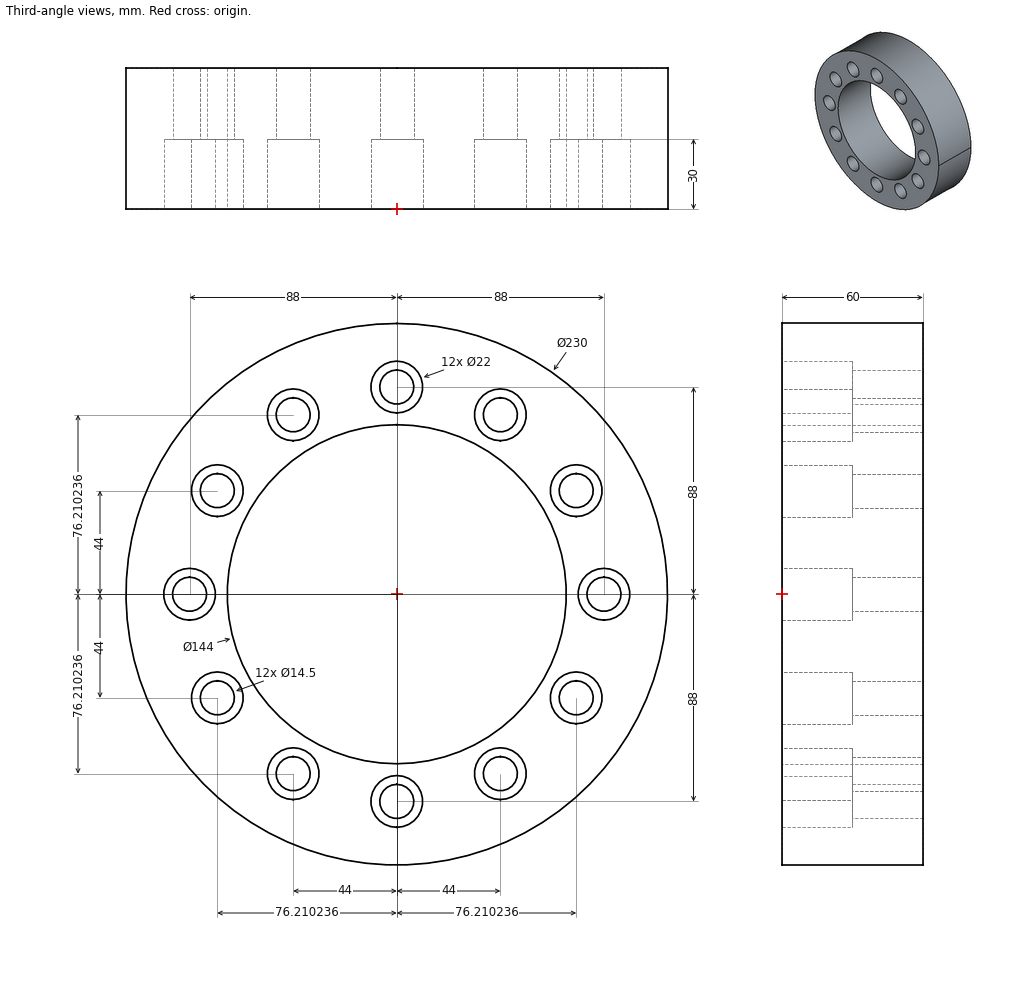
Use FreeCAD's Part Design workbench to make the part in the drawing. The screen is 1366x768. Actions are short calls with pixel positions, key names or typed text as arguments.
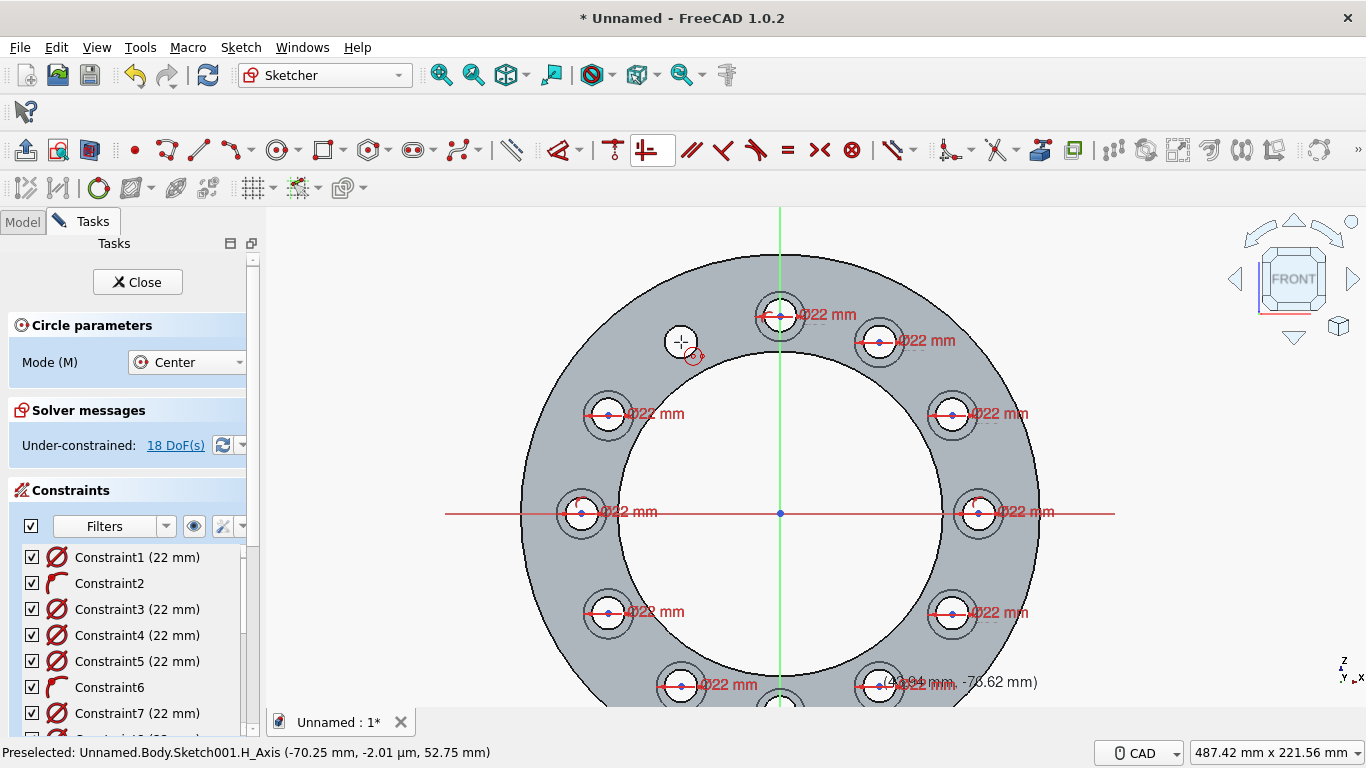
click(681, 342)
move(699, 324)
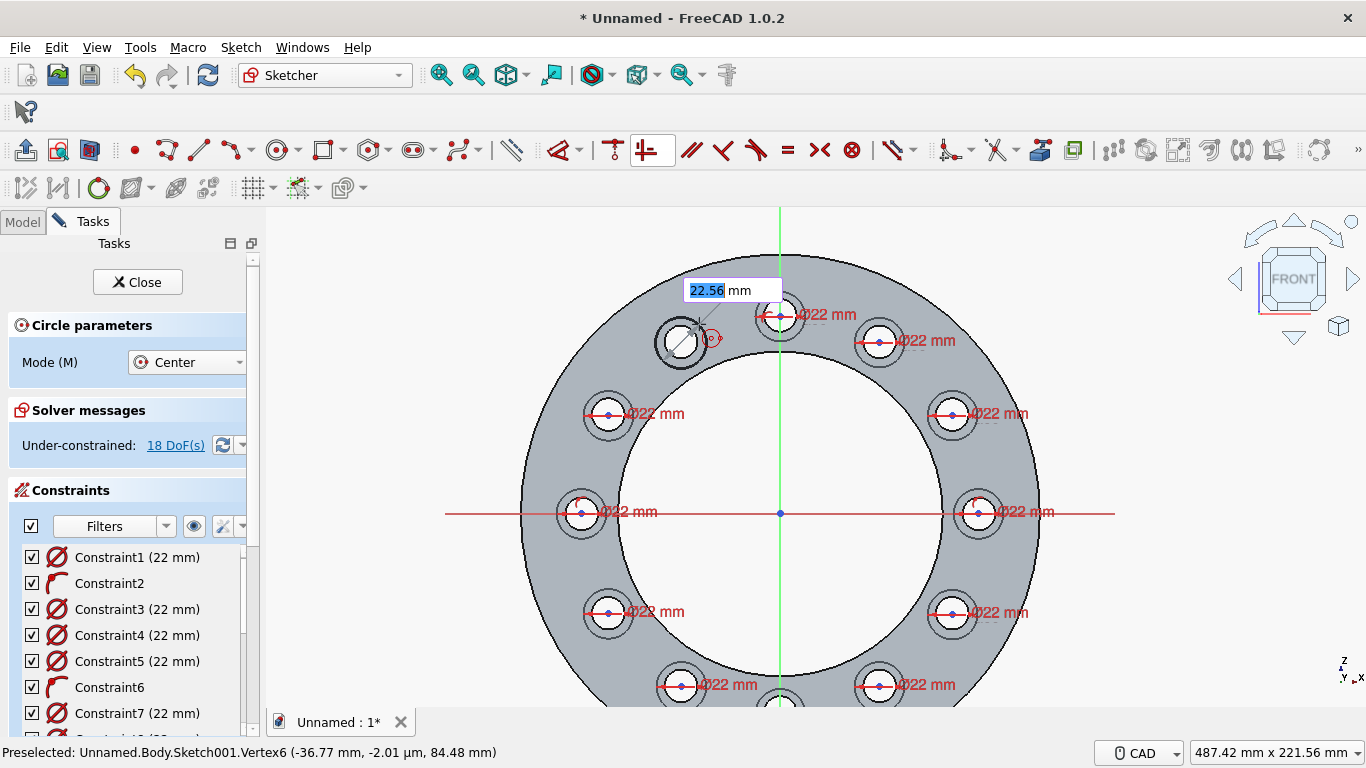
text(22)
key(Return)
key(Escape)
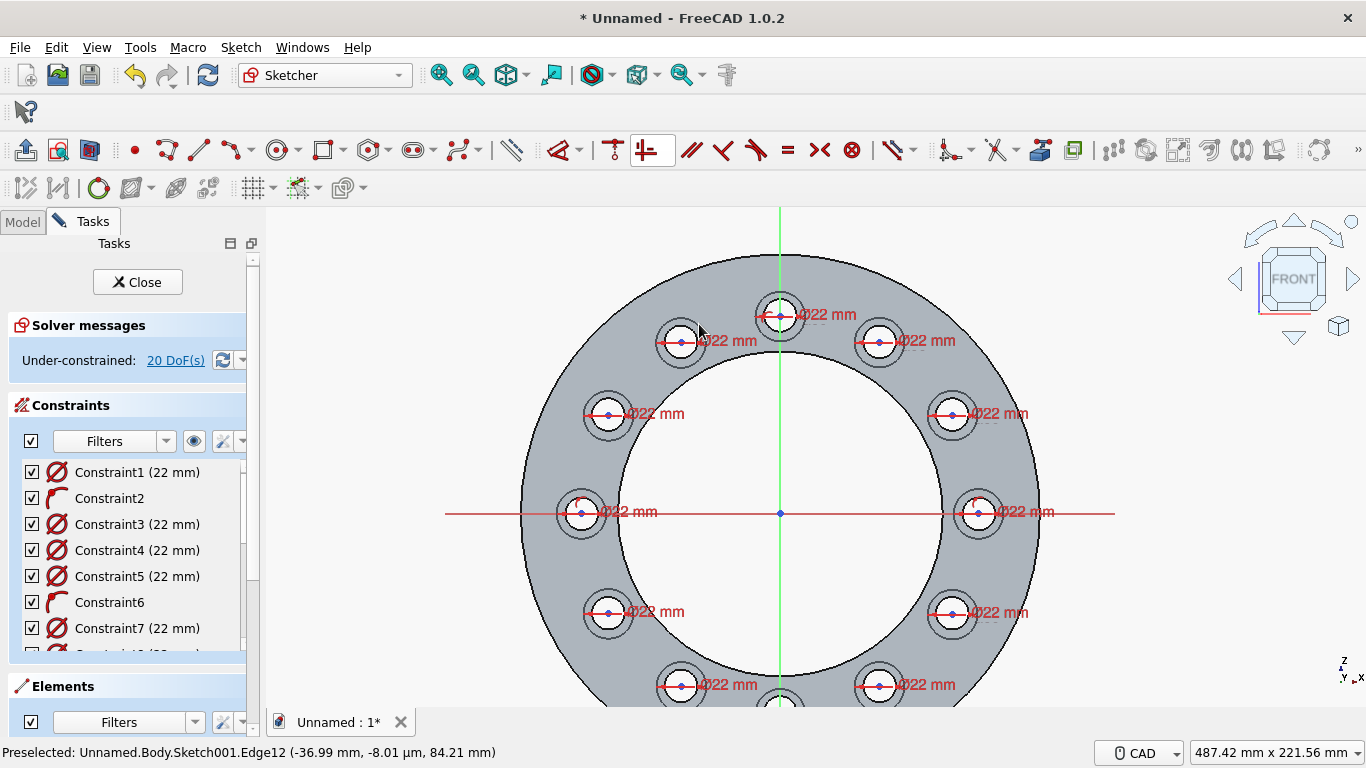
click(953, 416)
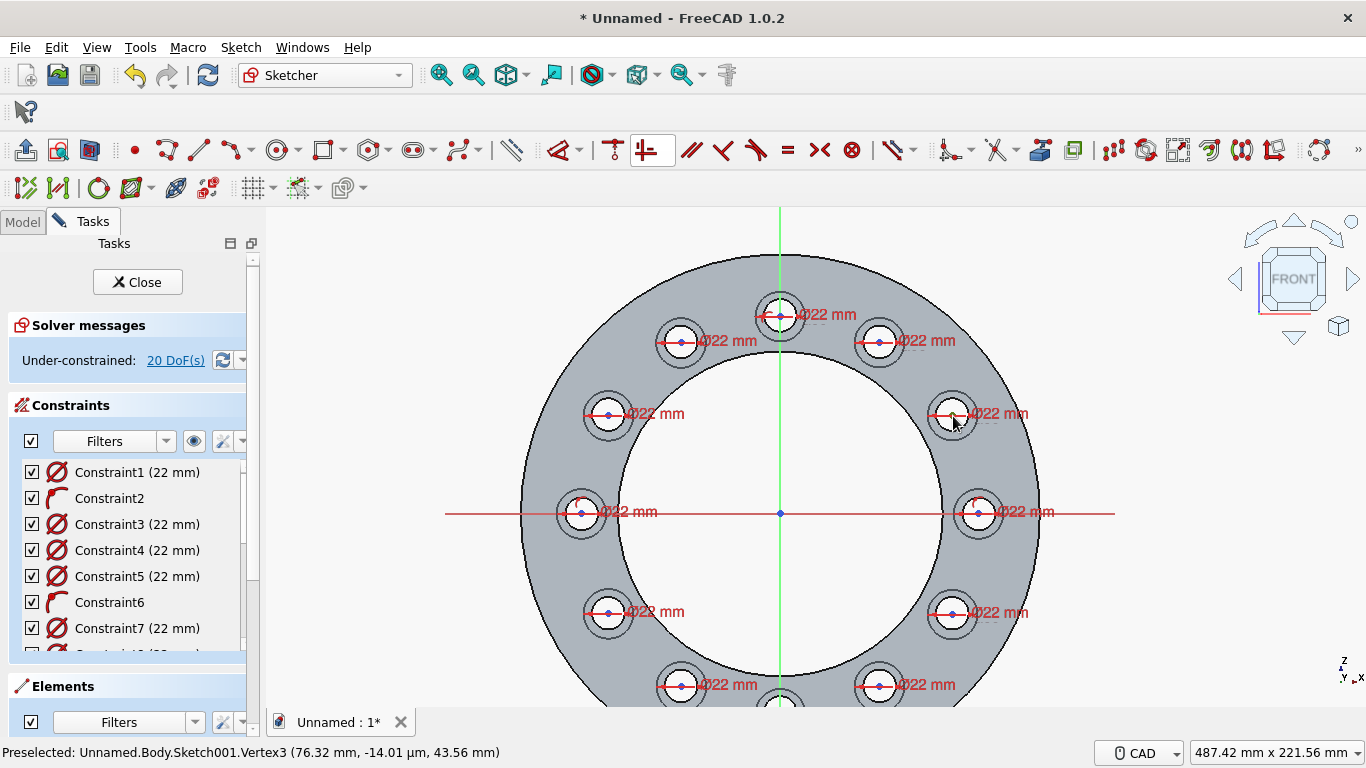
click(953, 615)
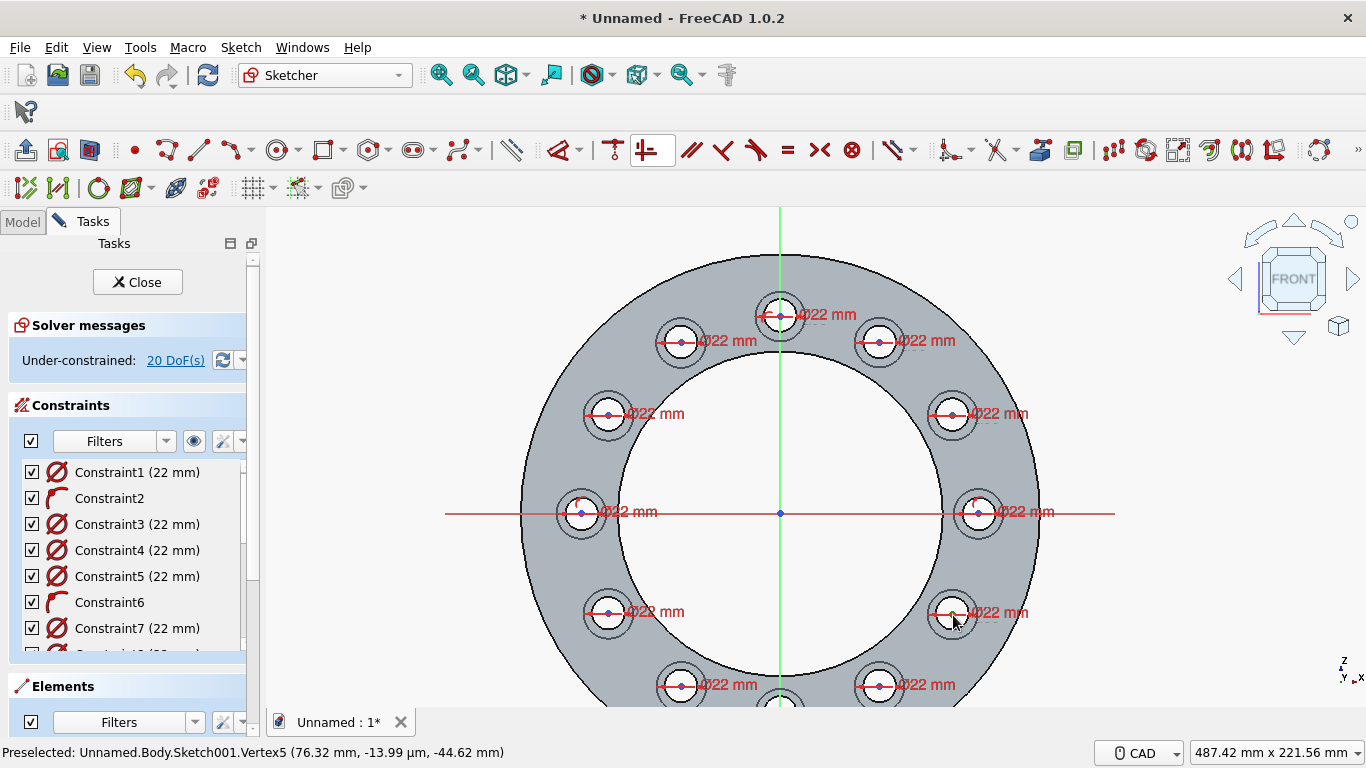
click(670, 150)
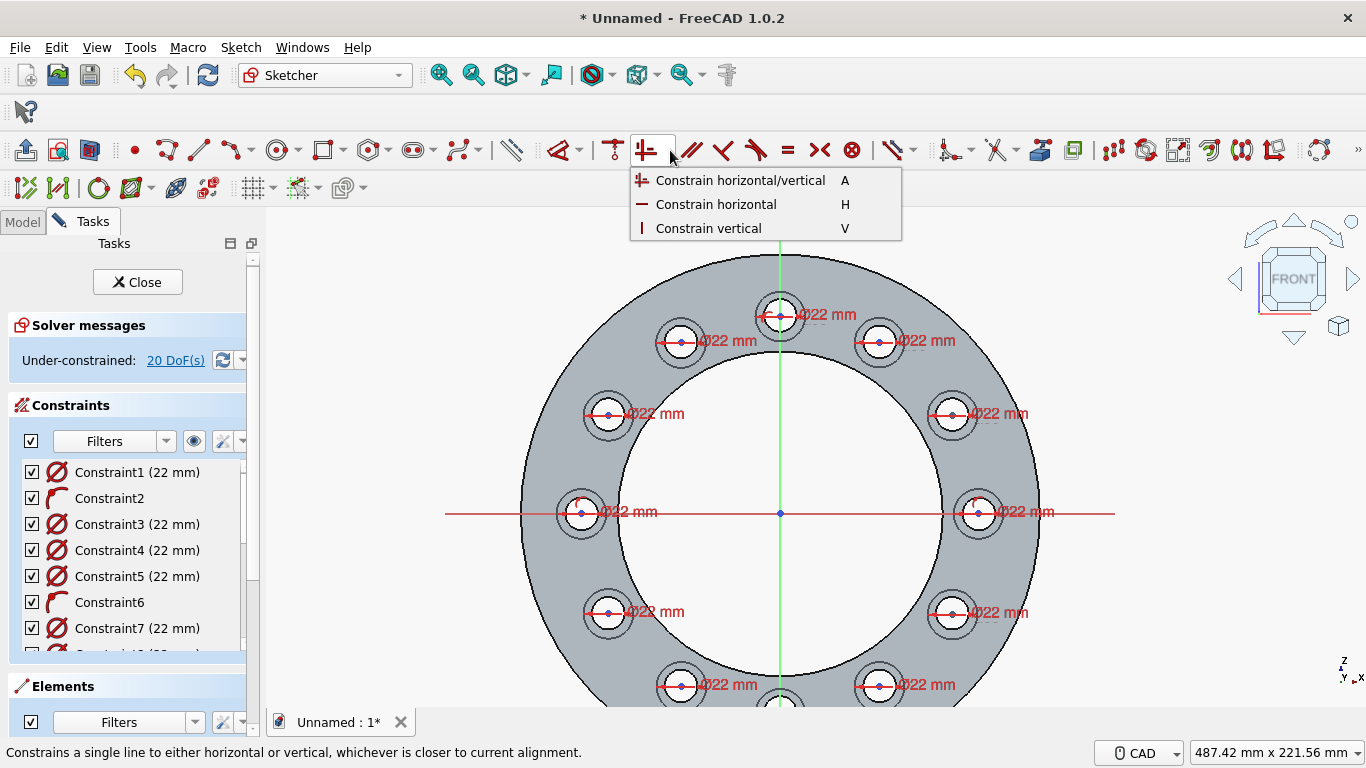
click(766, 228)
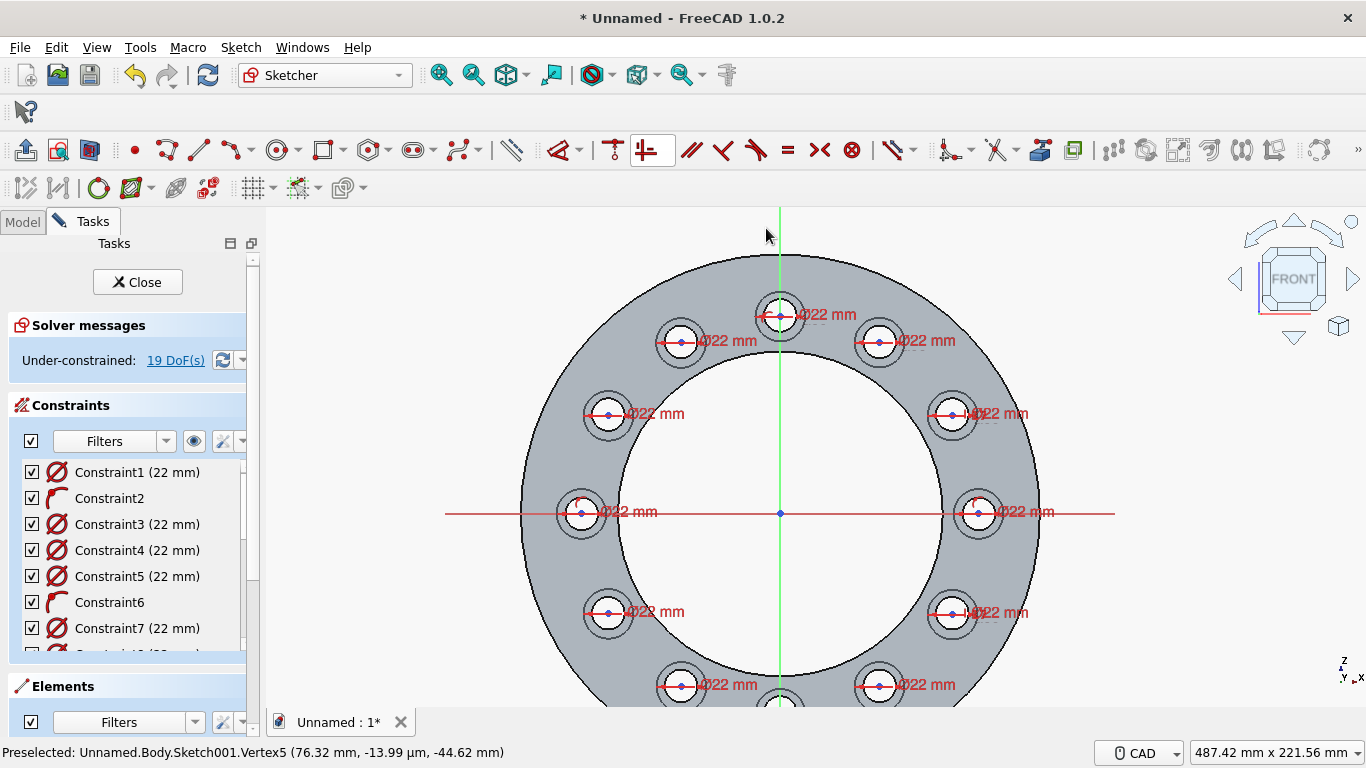
click(880, 343)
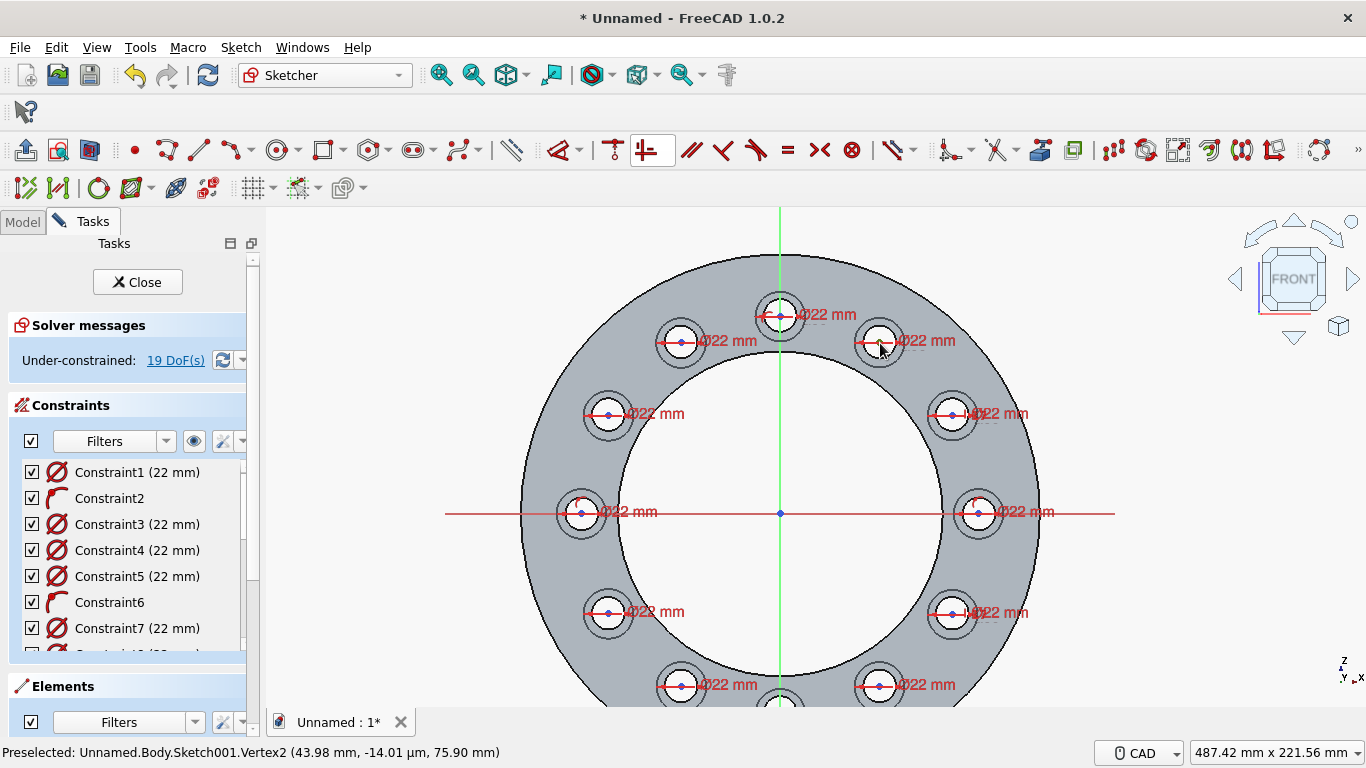
scroll(681, 341, down, 2)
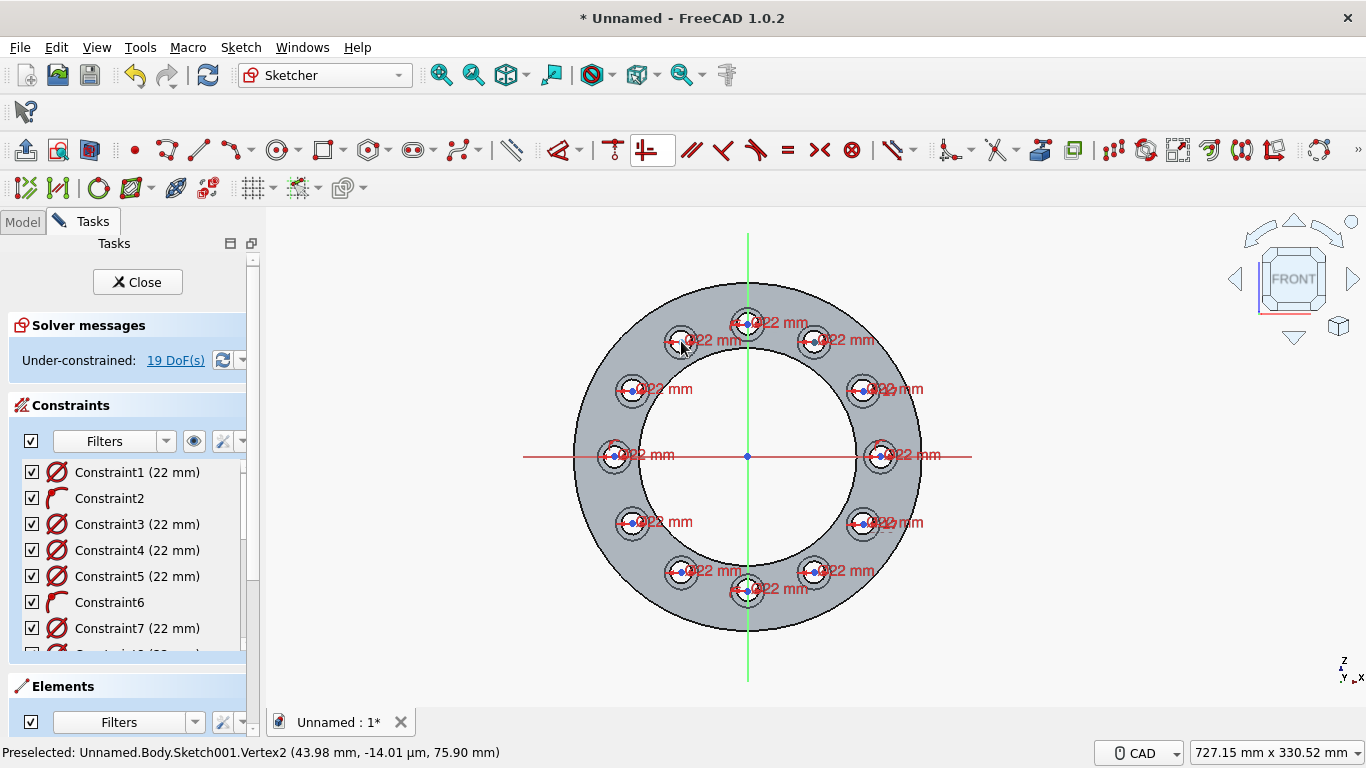
click(814, 573)